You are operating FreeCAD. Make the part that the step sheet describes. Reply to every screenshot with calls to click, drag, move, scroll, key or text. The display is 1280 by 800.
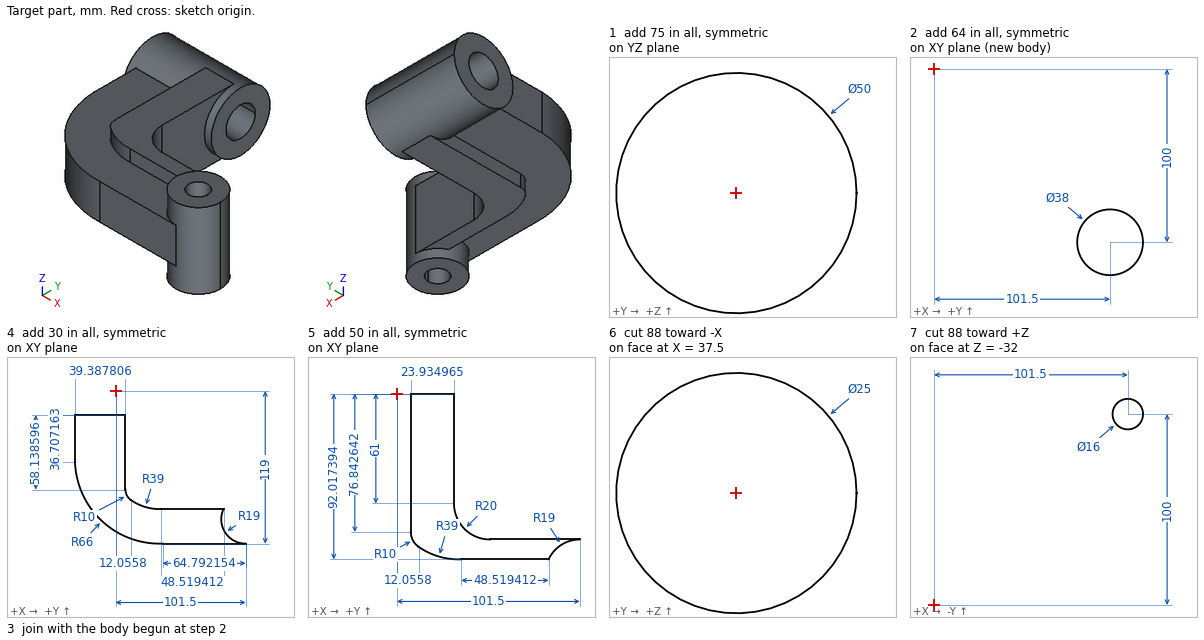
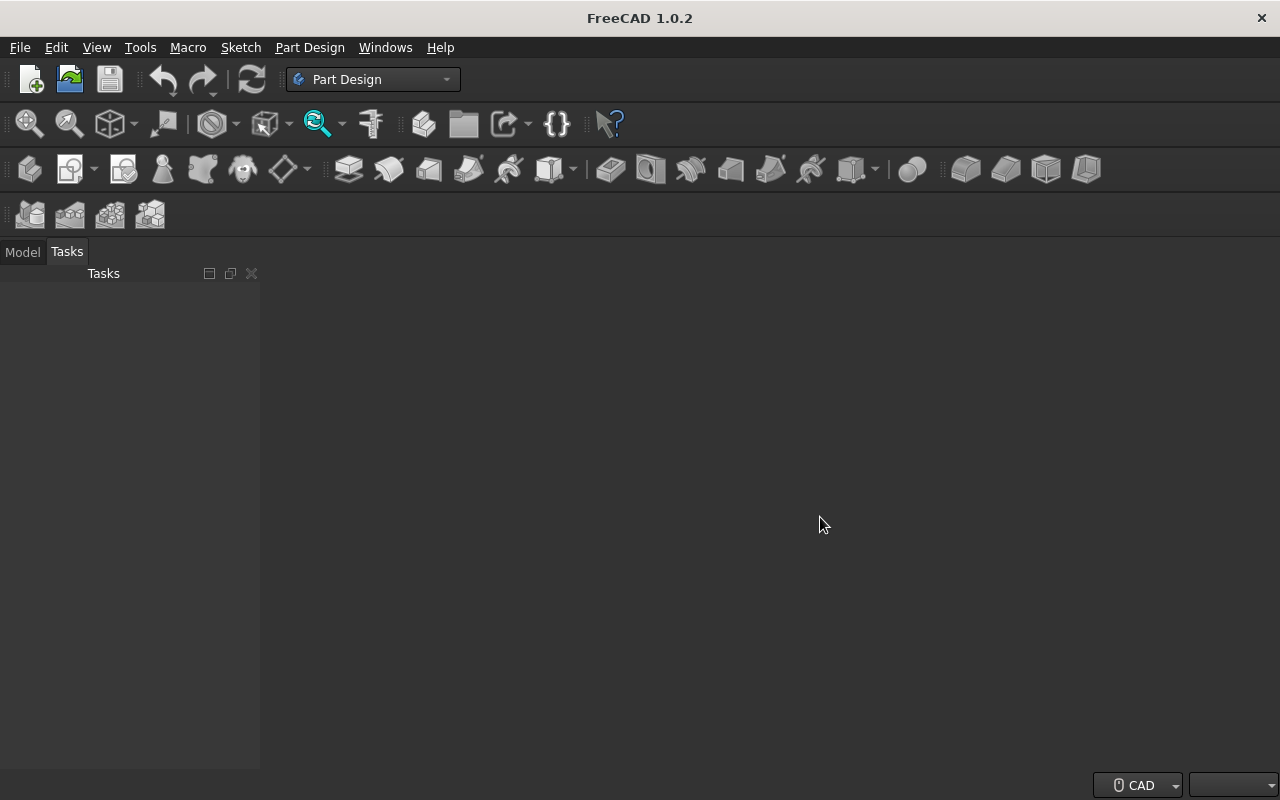
click(30, 80)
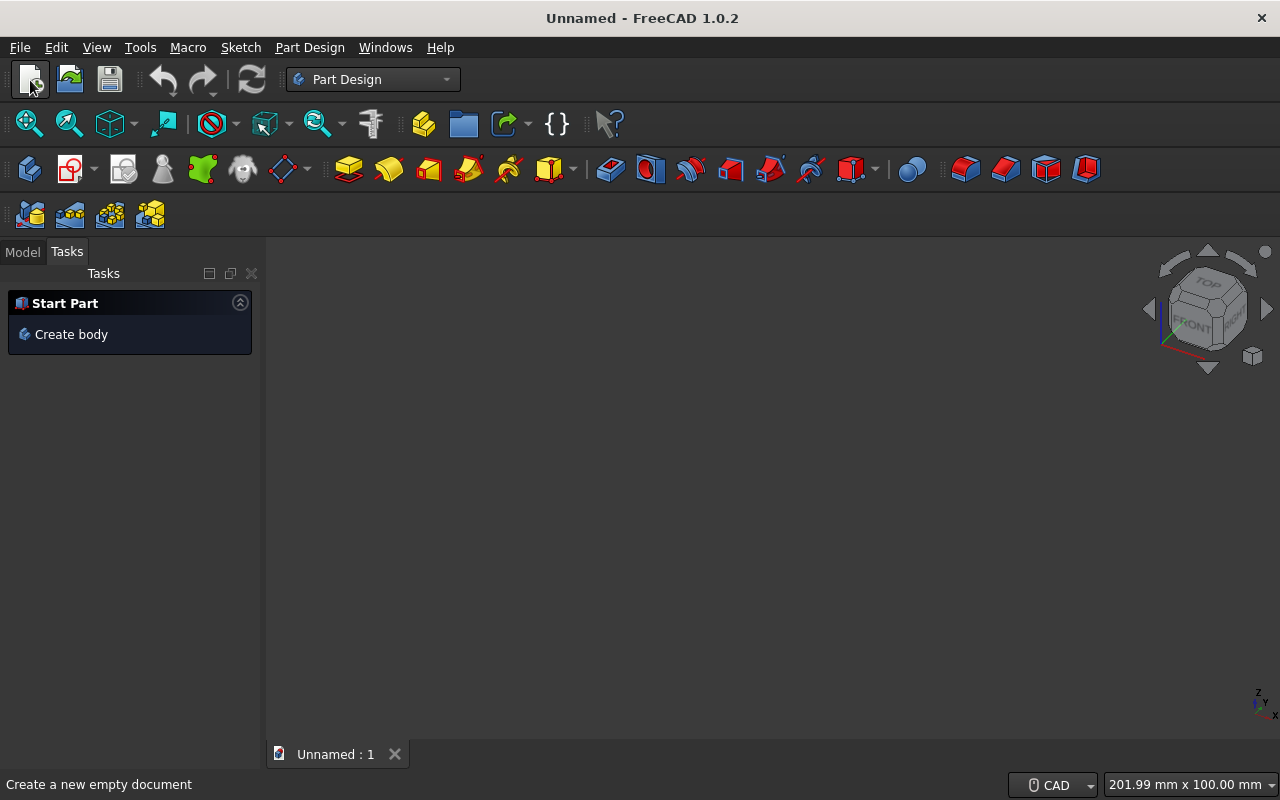
click(70, 170)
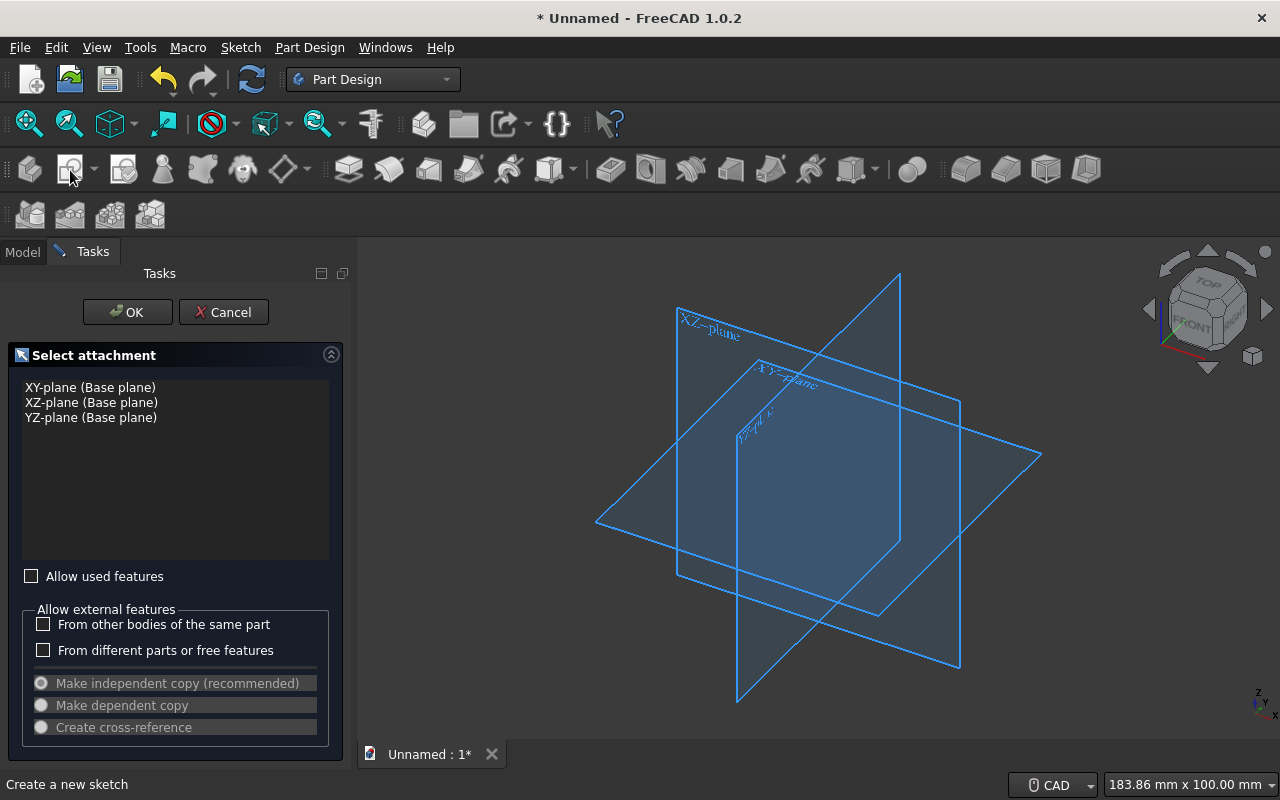
click(82, 418)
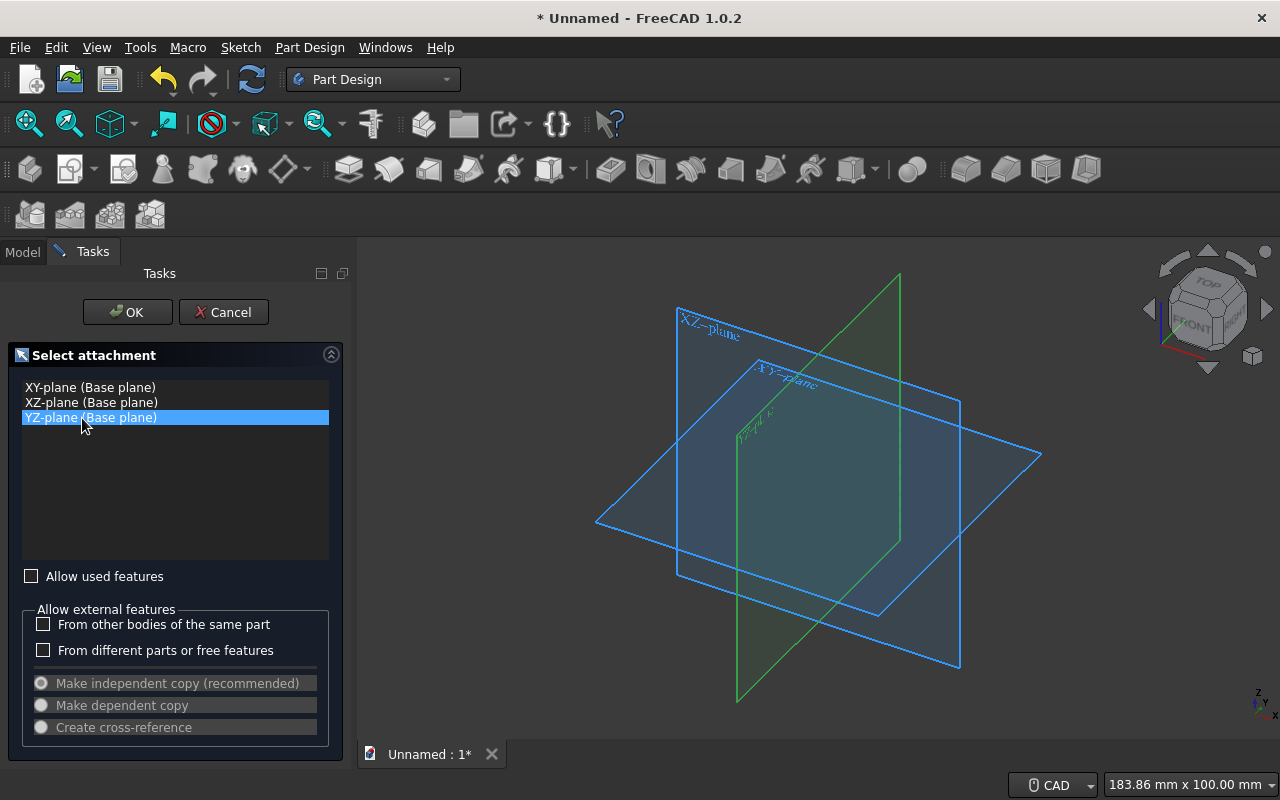
click(128, 312)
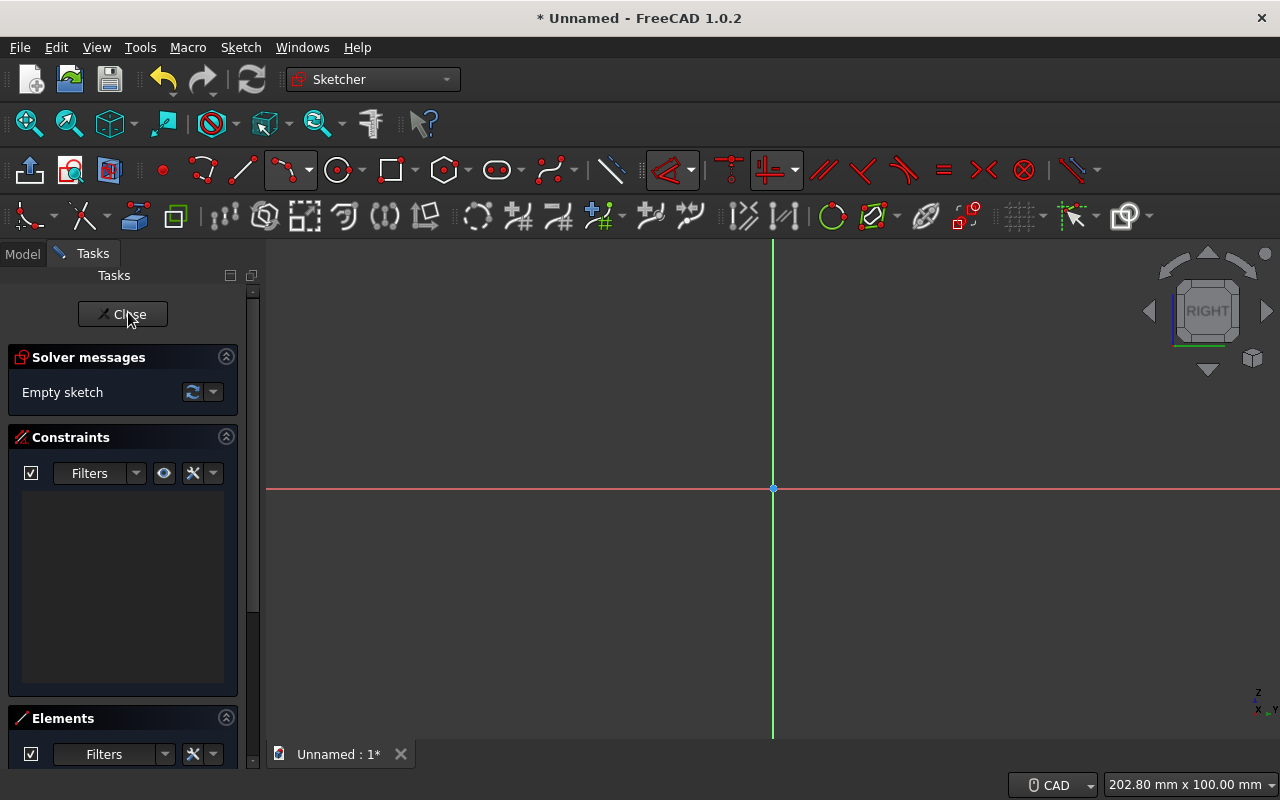
click(338, 170)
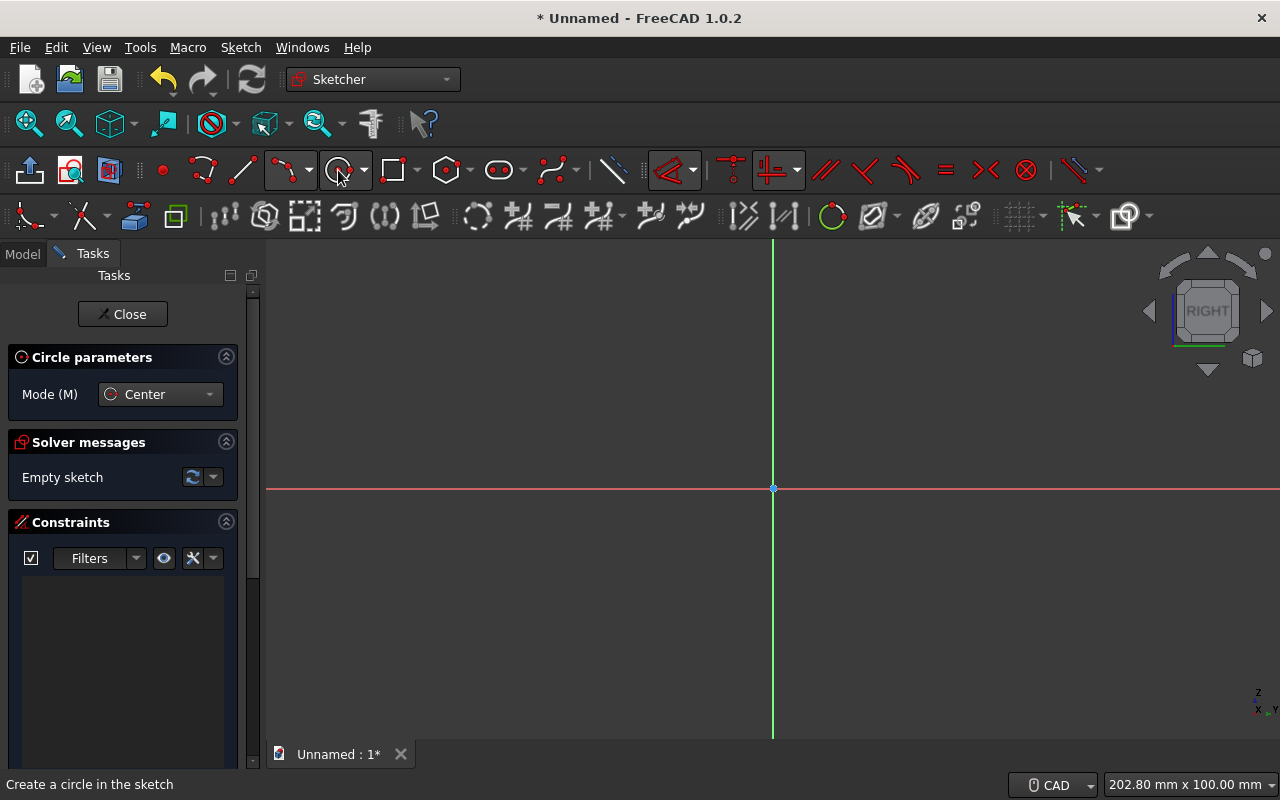
click(773, 489)
click(861, 401)
key(Escape)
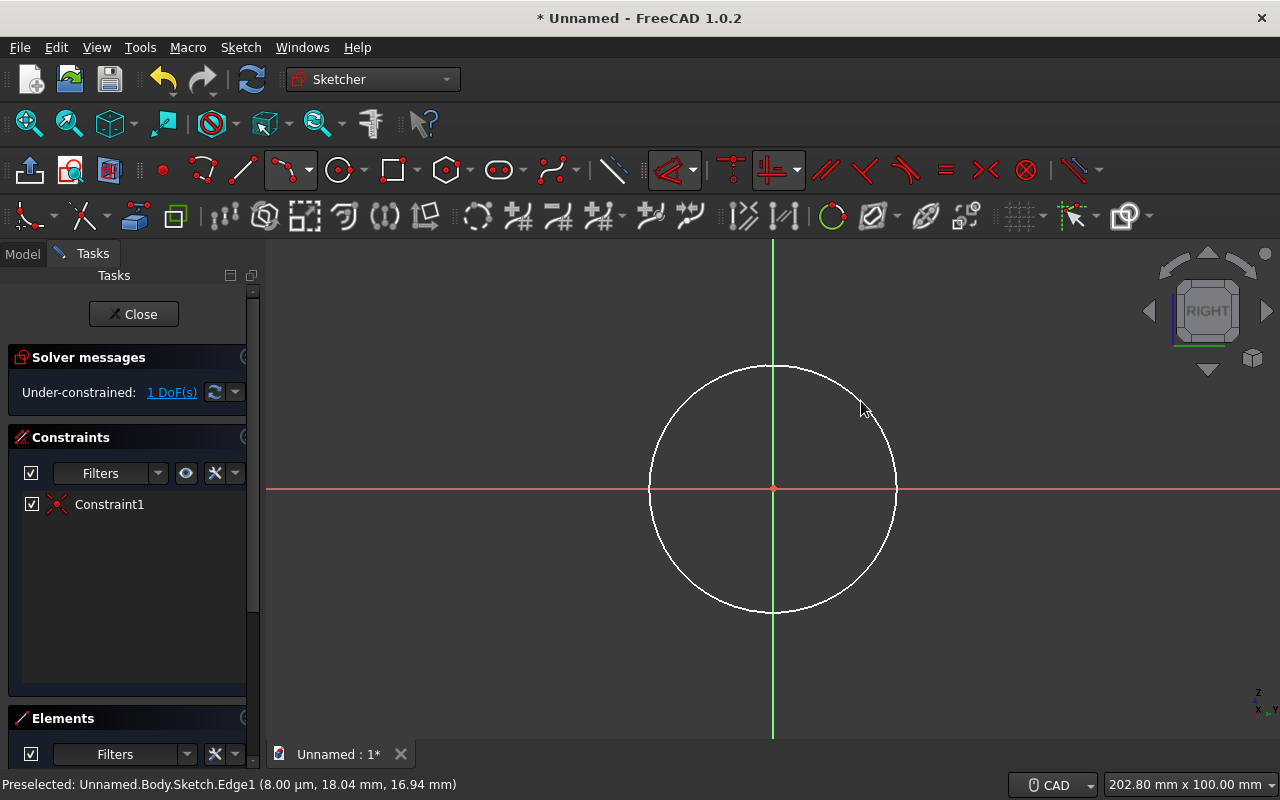
click(668, 170)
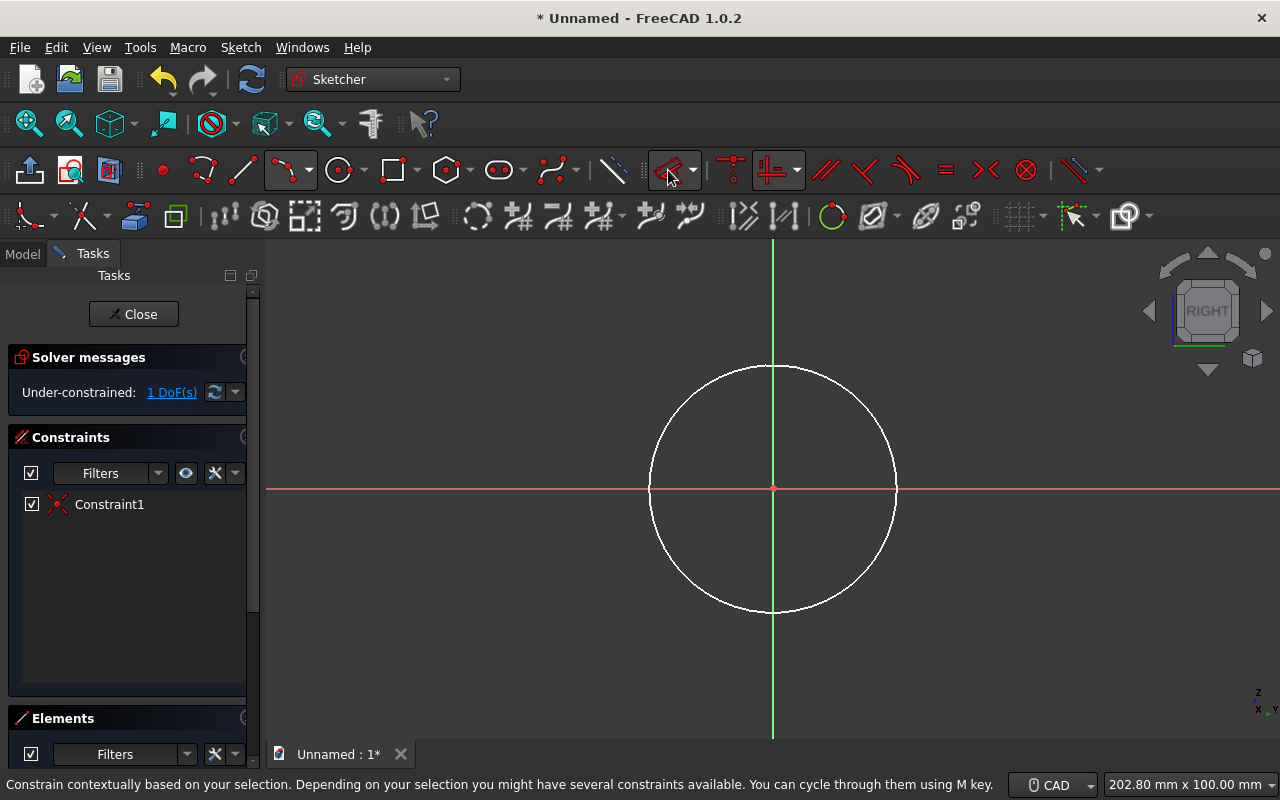
click(860, 401)
click(882, 378)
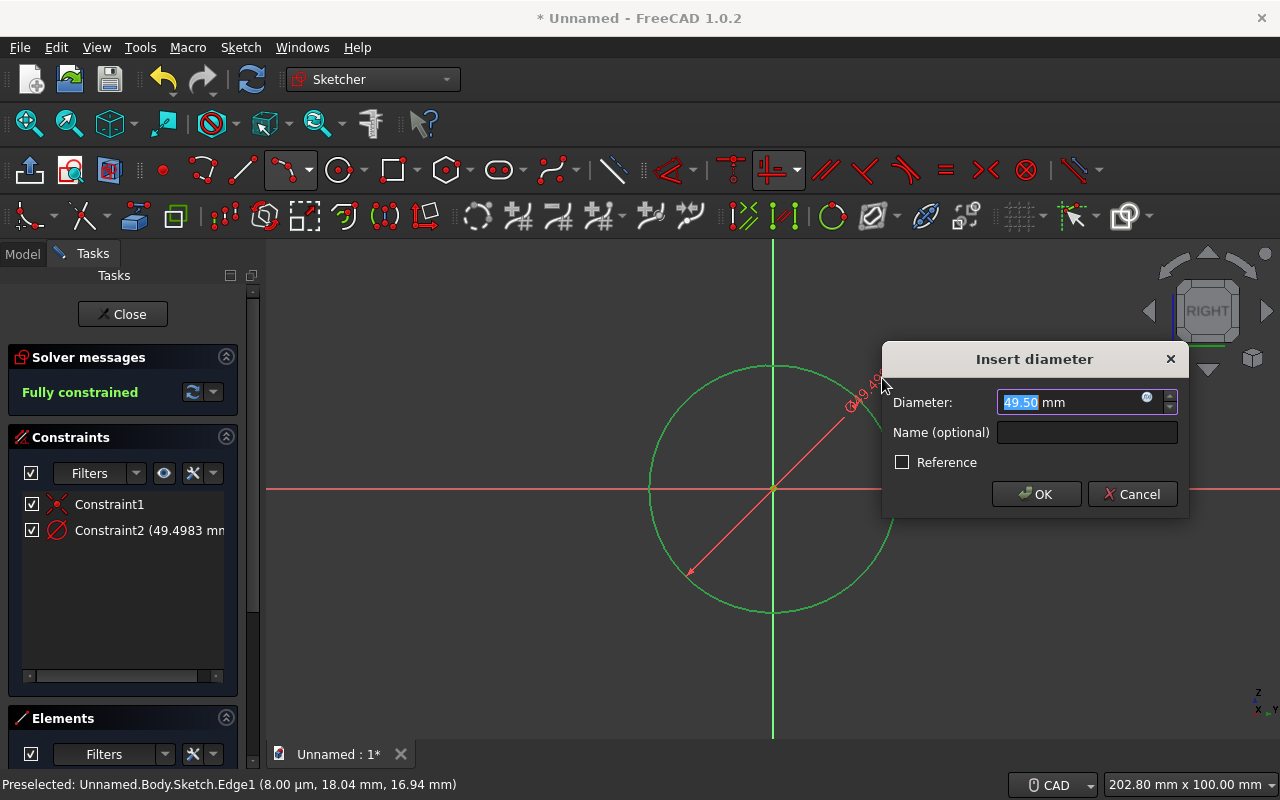
text(50)
key(Return)
key(Escape)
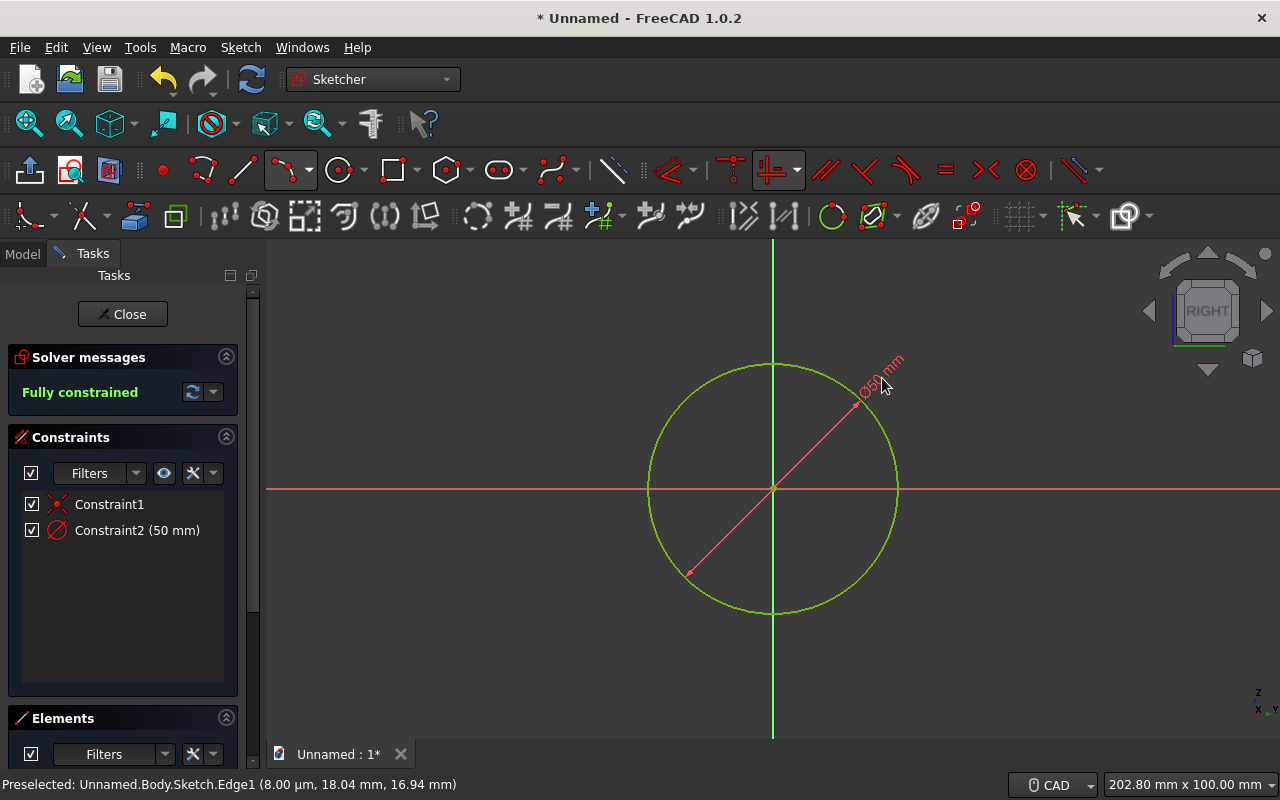
click(123, 314)